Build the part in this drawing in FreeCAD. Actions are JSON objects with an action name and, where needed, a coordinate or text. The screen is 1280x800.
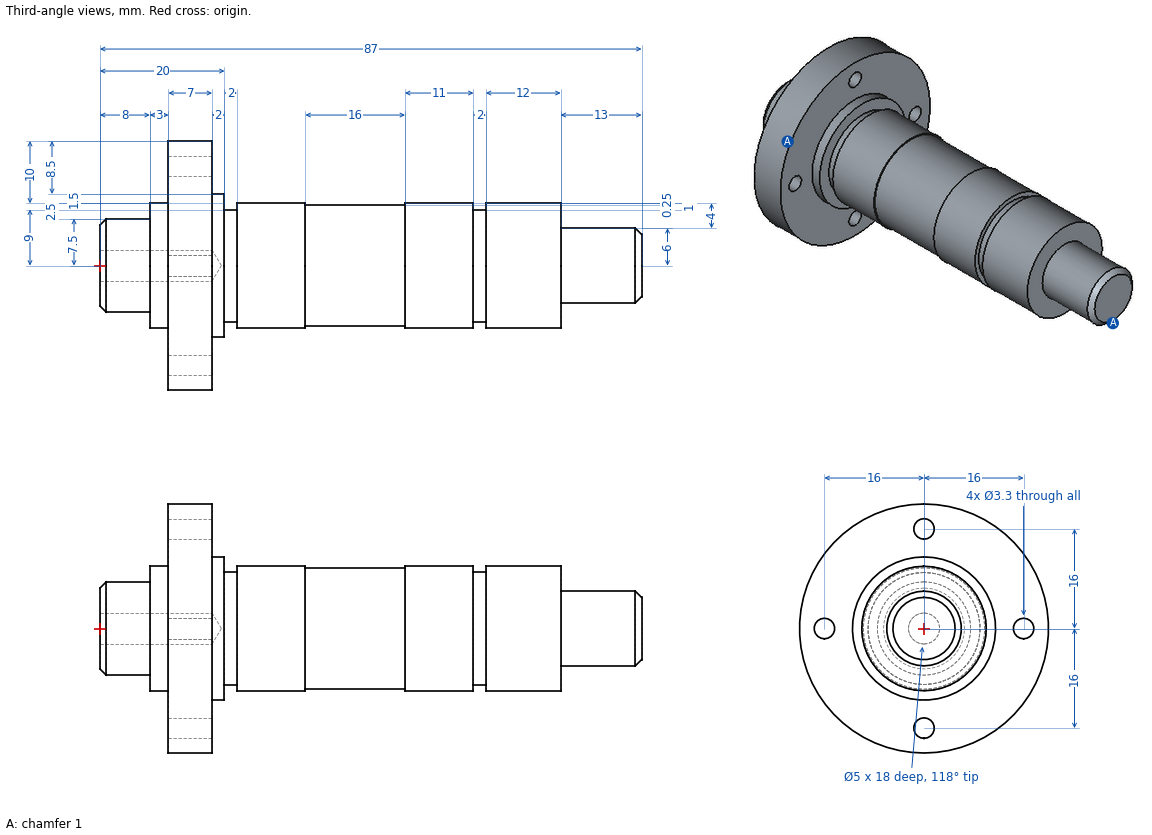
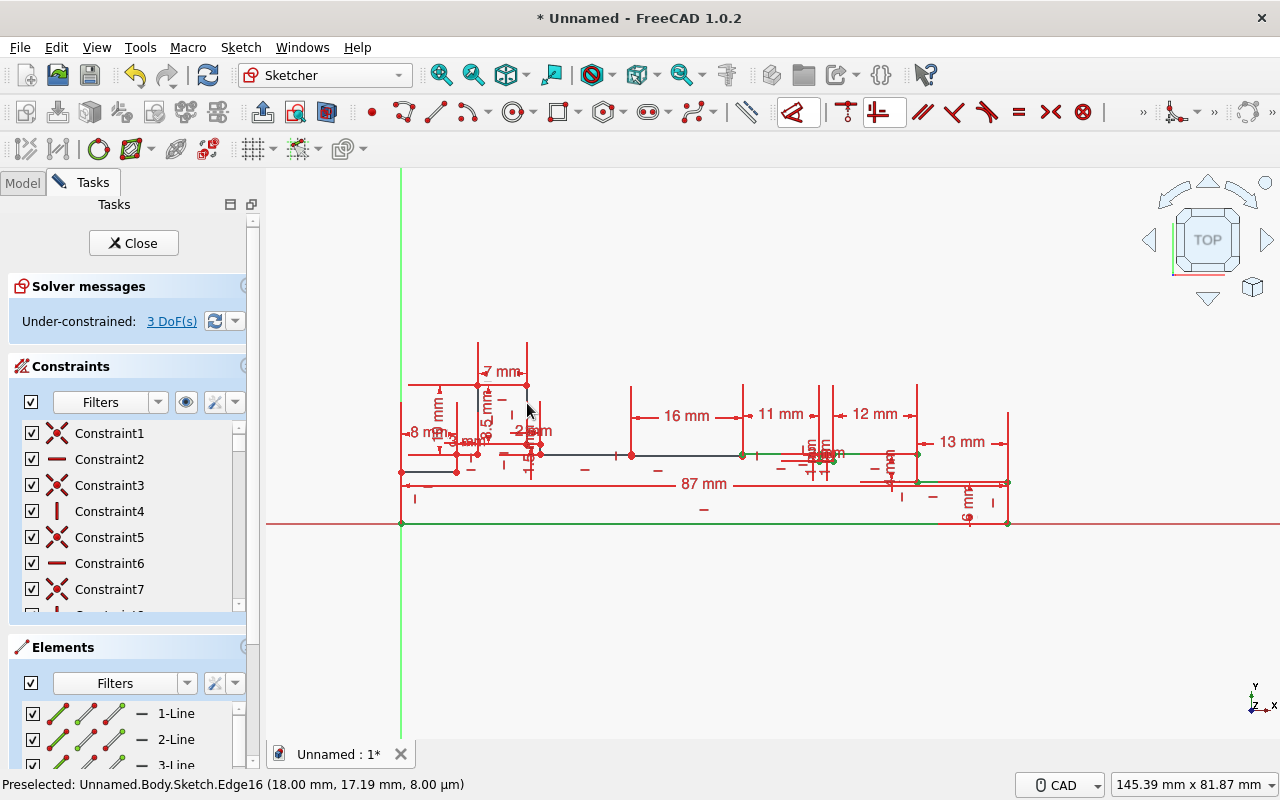
{"action": "scroll", "coordinate": [457, 464], "scroll_direction": "up", "scroll_amount": 5}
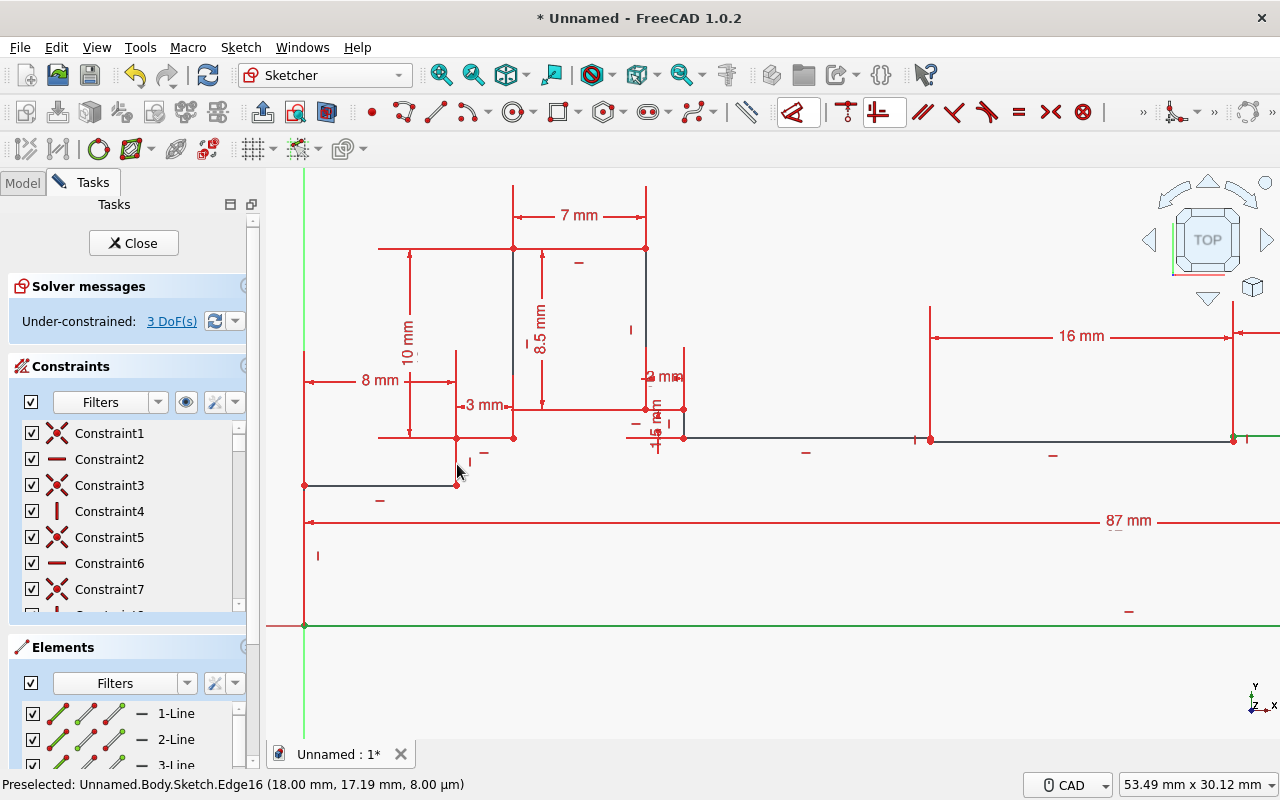
{"action": "left_click", "coordinate": [456, 462]}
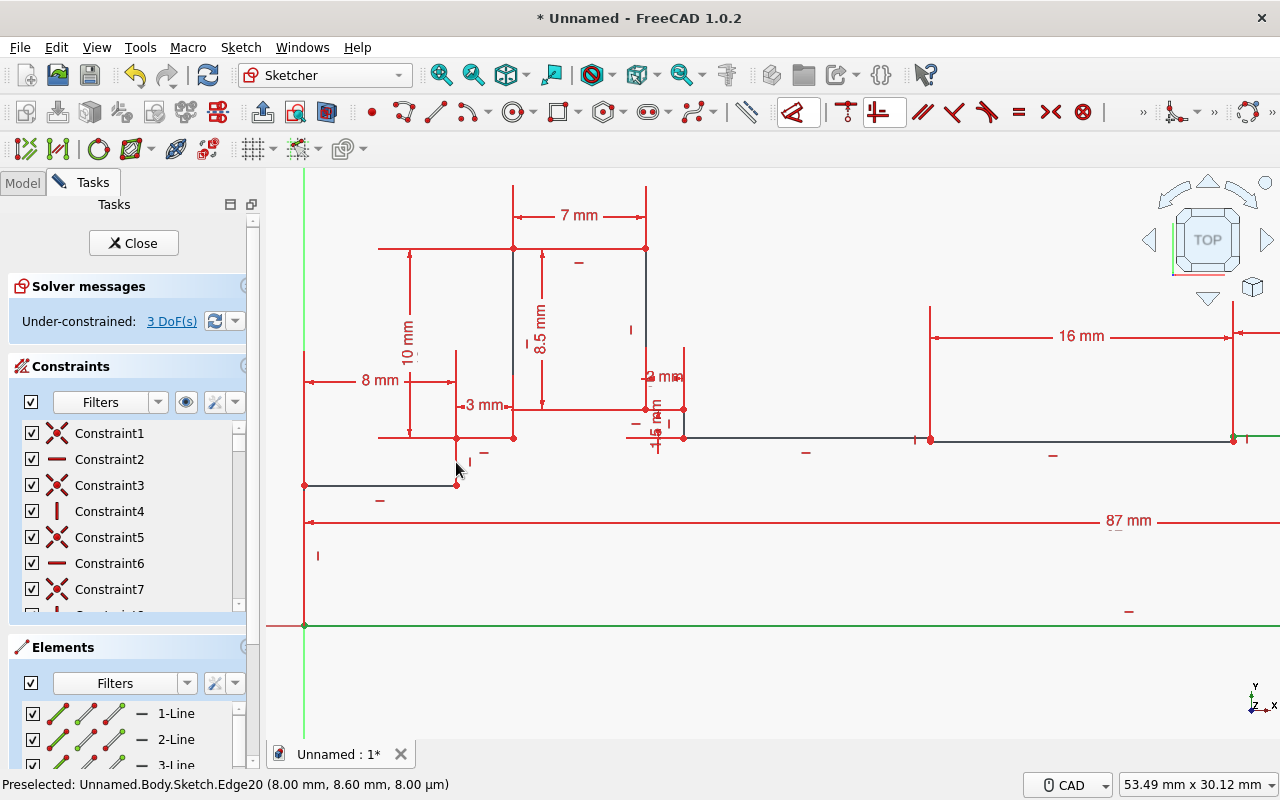
{"action": "key", "text": "i"}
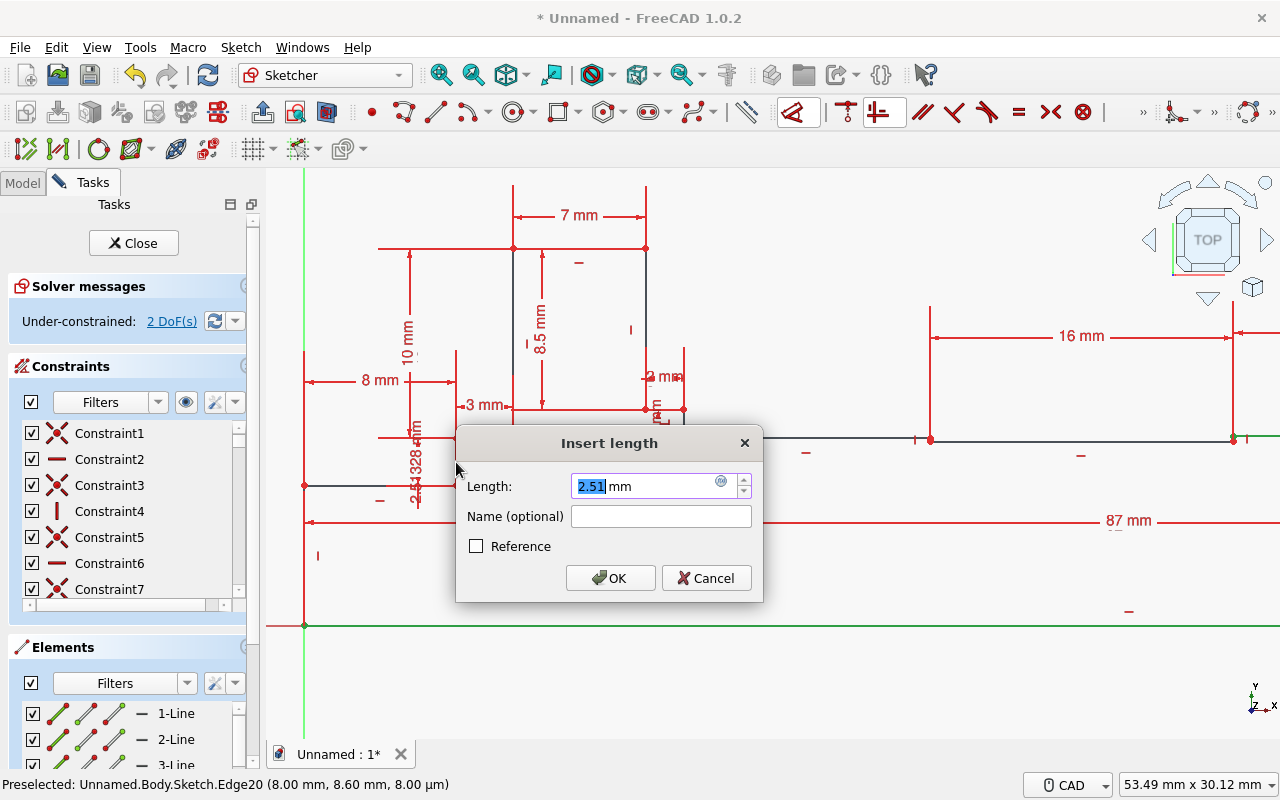
{"action": "type", "text": "2.5"}
{"action": "key", "text": "Return"}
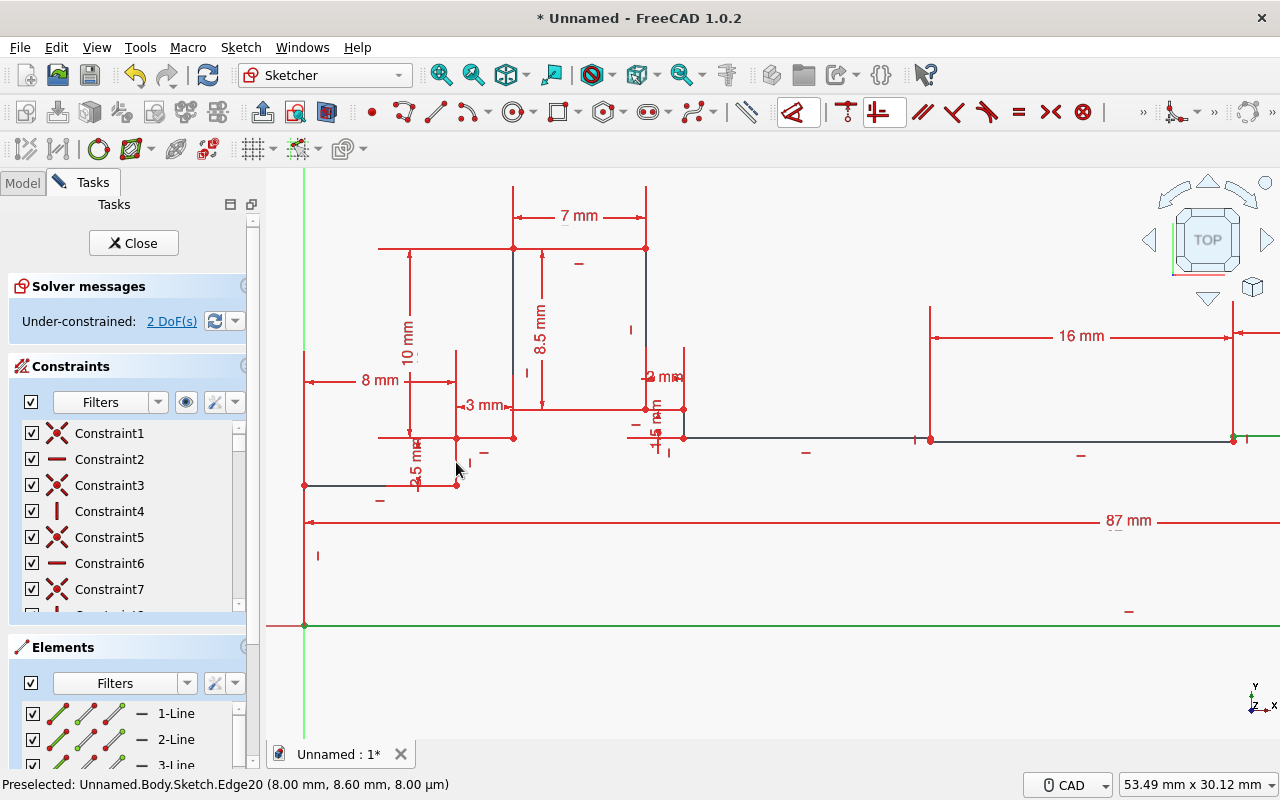
{"action": "left_click", "coordinate": [304, 528]}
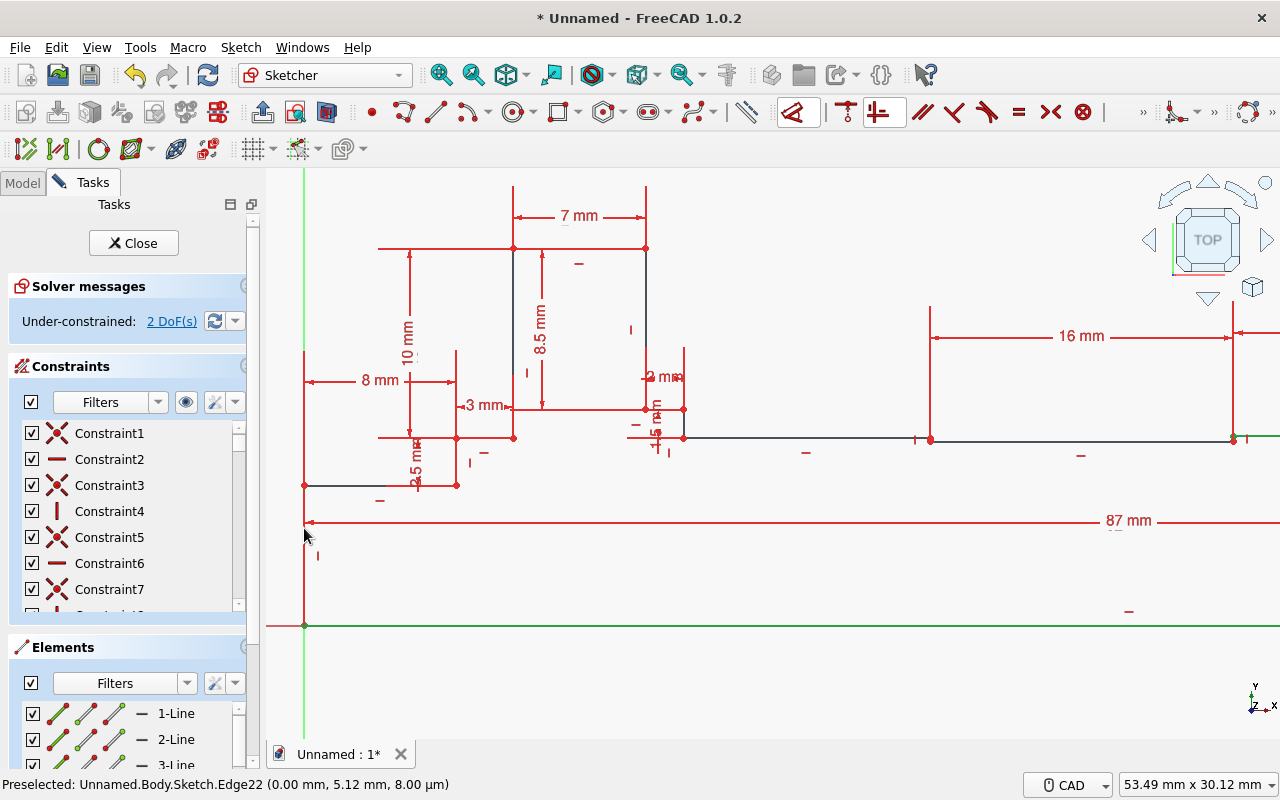
{"action": "key", "text": "i"}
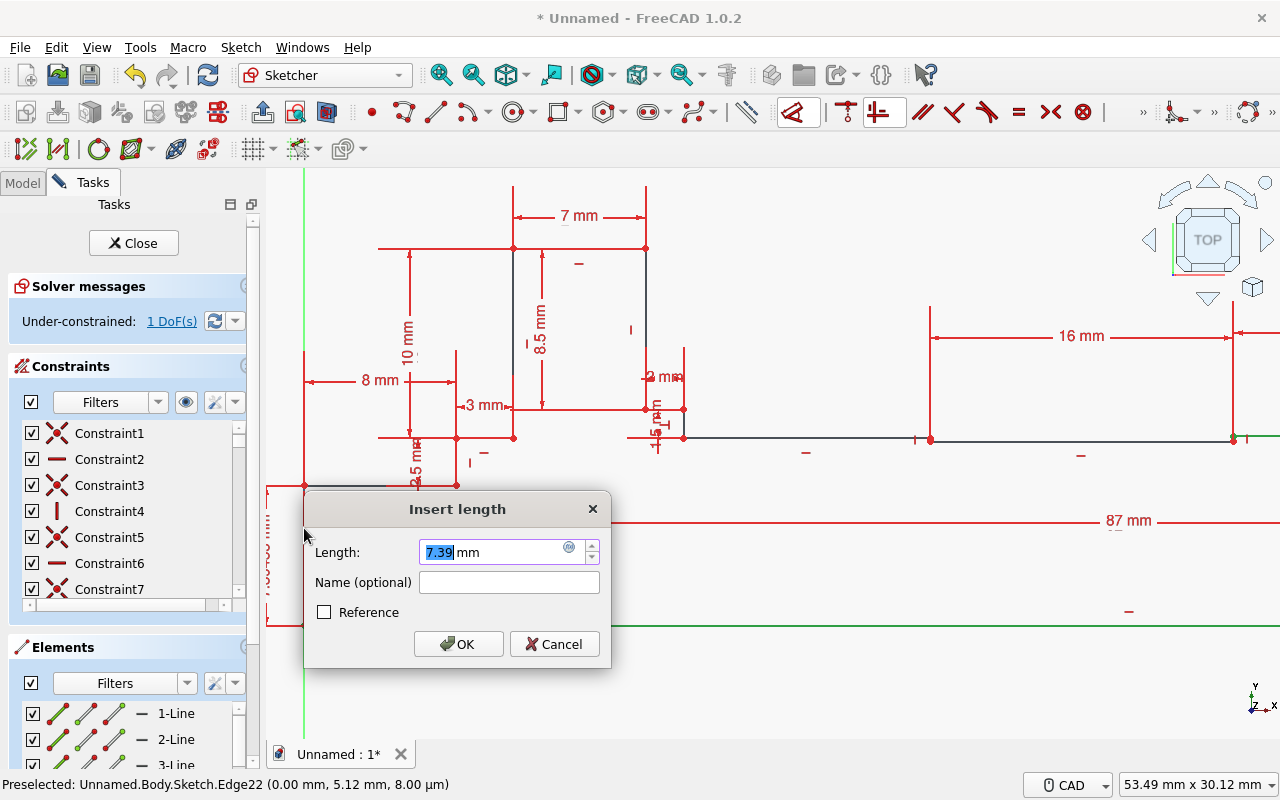
{"action": "type", "text": "7.5"}
{"action": "key", "text": "Return"}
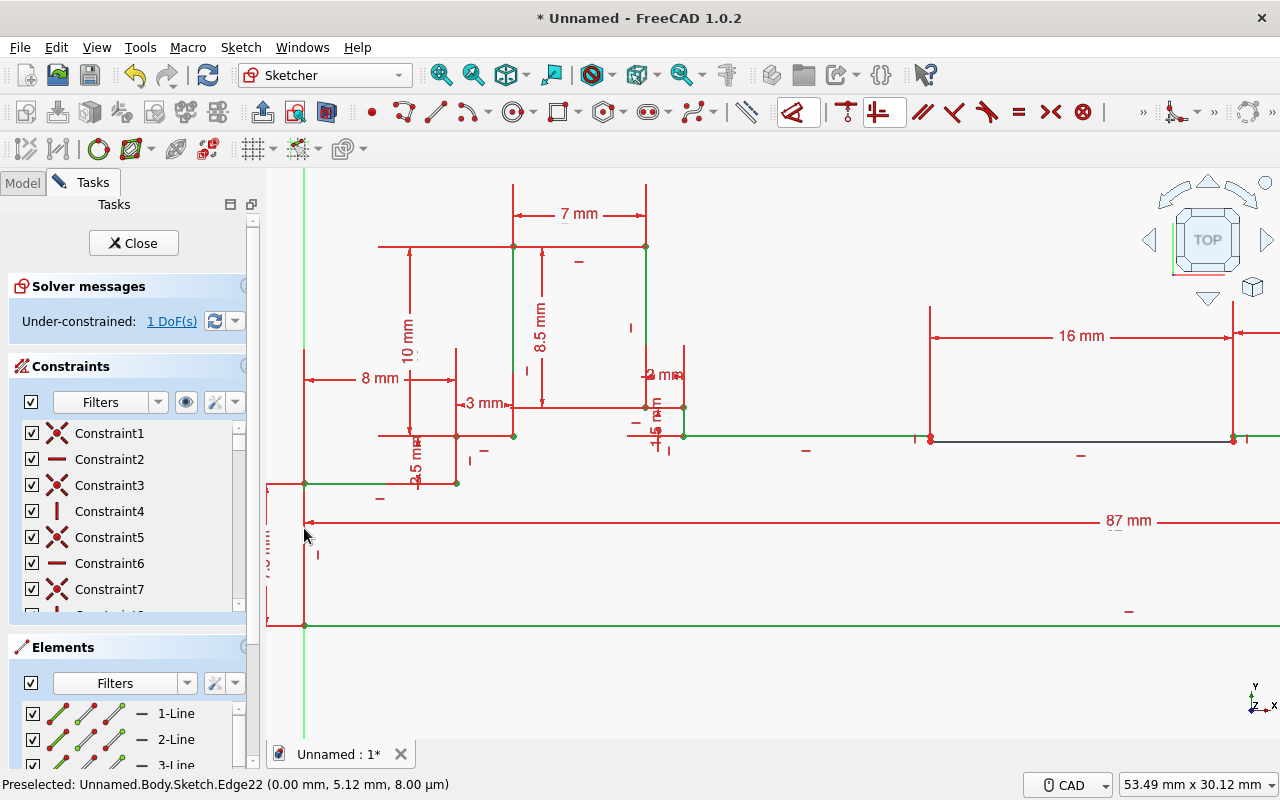
{"action": "scroll", "coordinate": [457, 463], "scroll_direction": "down", "scroll_amount": 5}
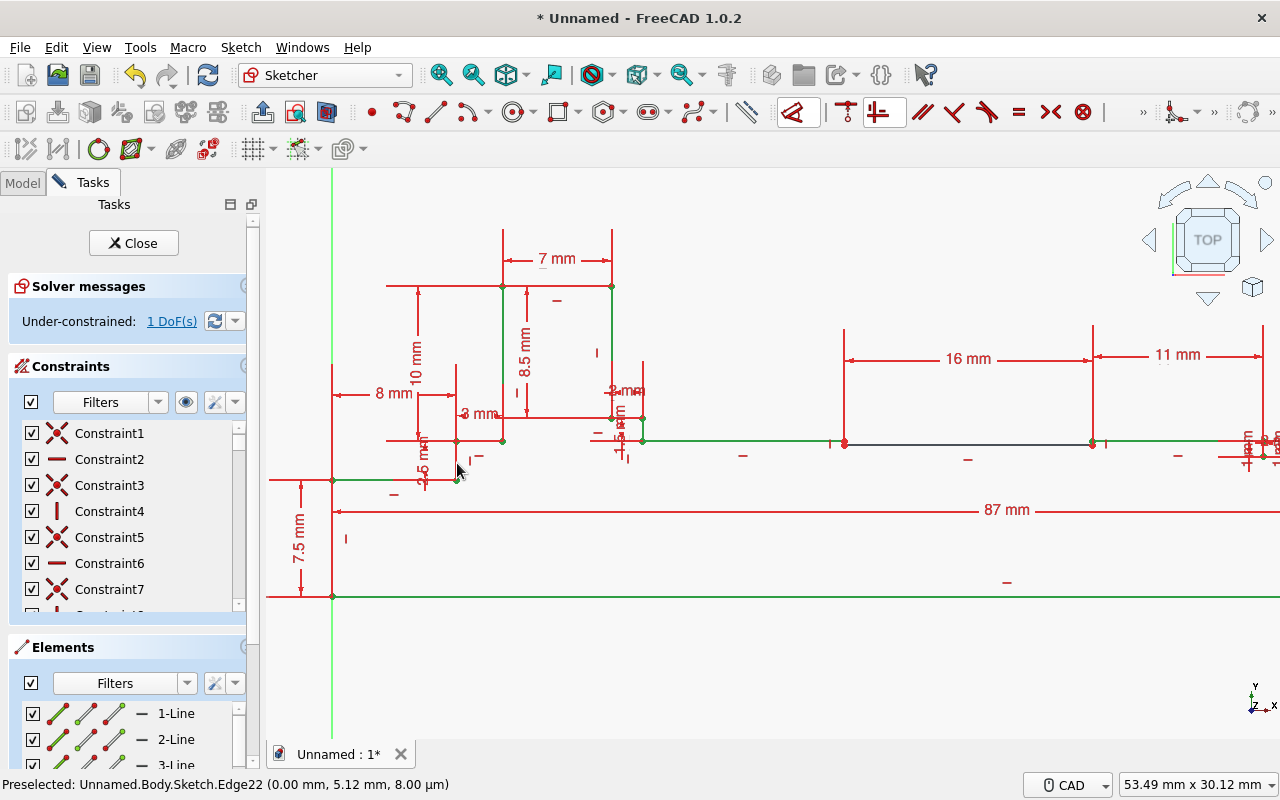
{"action": "scroll", "coordinate": [743, 454], "scroll_direction": "up", "scroll_amount": 16}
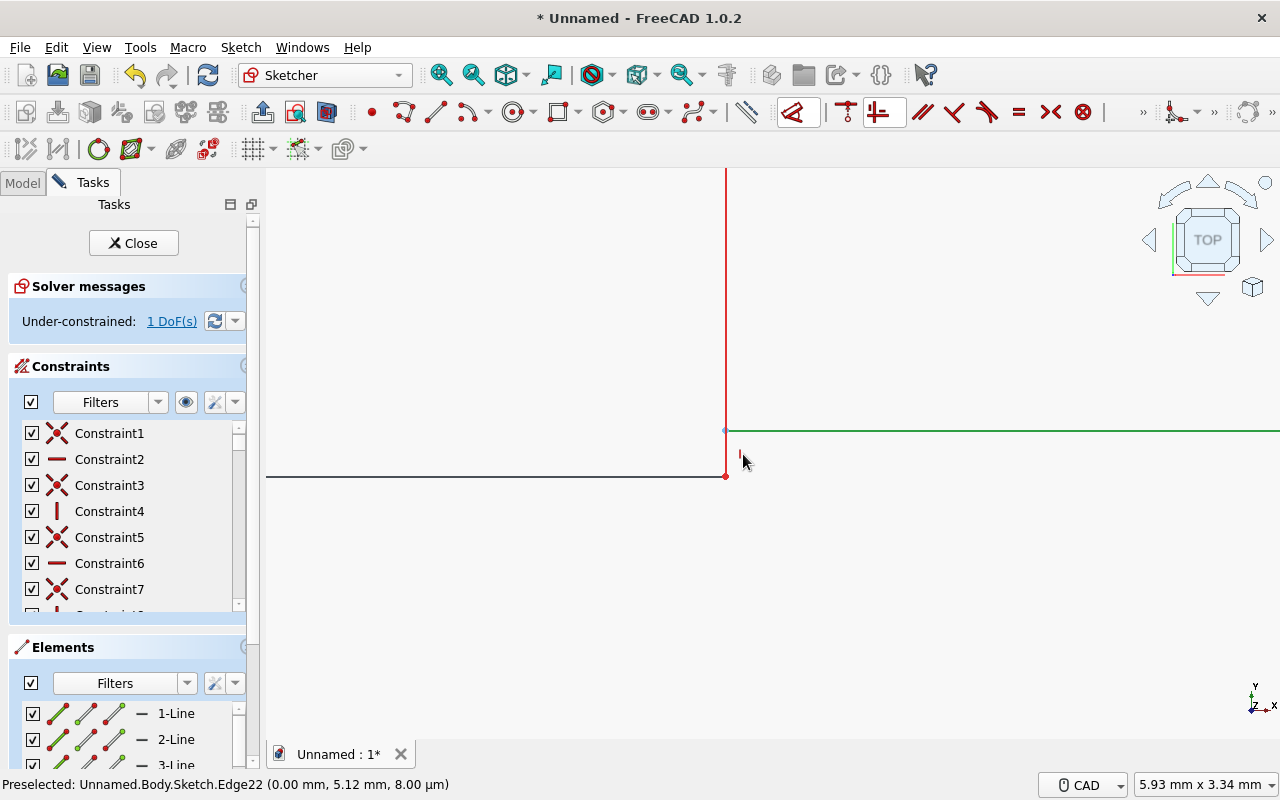
{"action": "left_click", "coordinate": [726, 454]}